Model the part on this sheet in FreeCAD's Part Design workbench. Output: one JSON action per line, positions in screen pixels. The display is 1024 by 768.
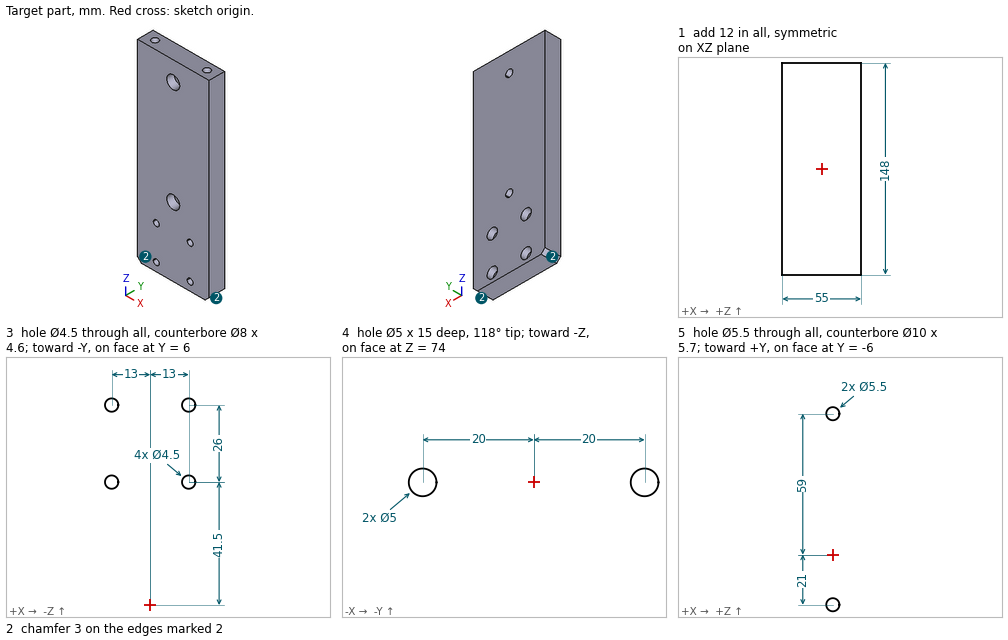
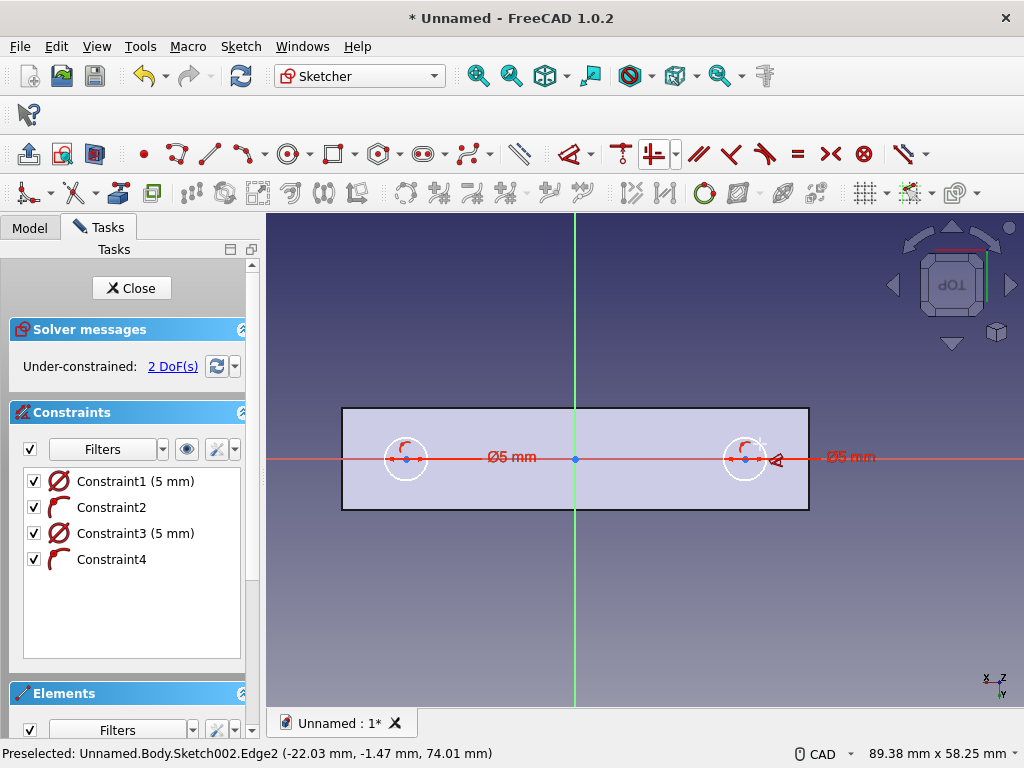
{"action": "left_click", "coordinate": [406, 459]}
{"action": "left_click", "coordinate": [491, 493]}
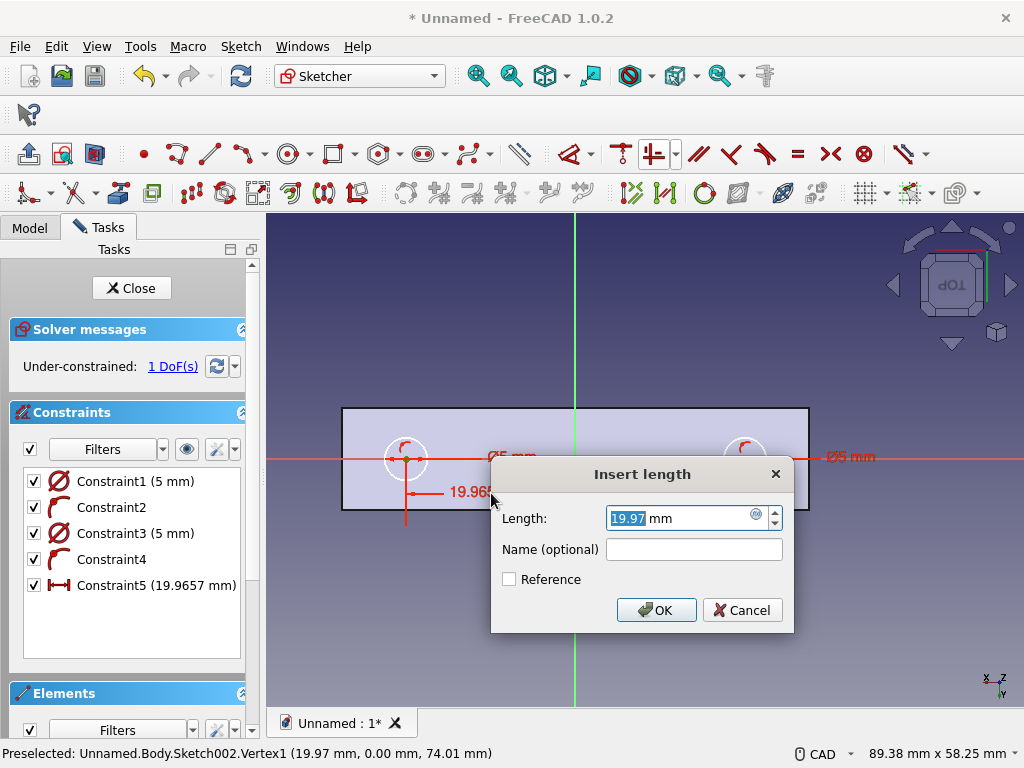
{"action": "type", "text": "20"}
{"action": "key", "text": "Return"}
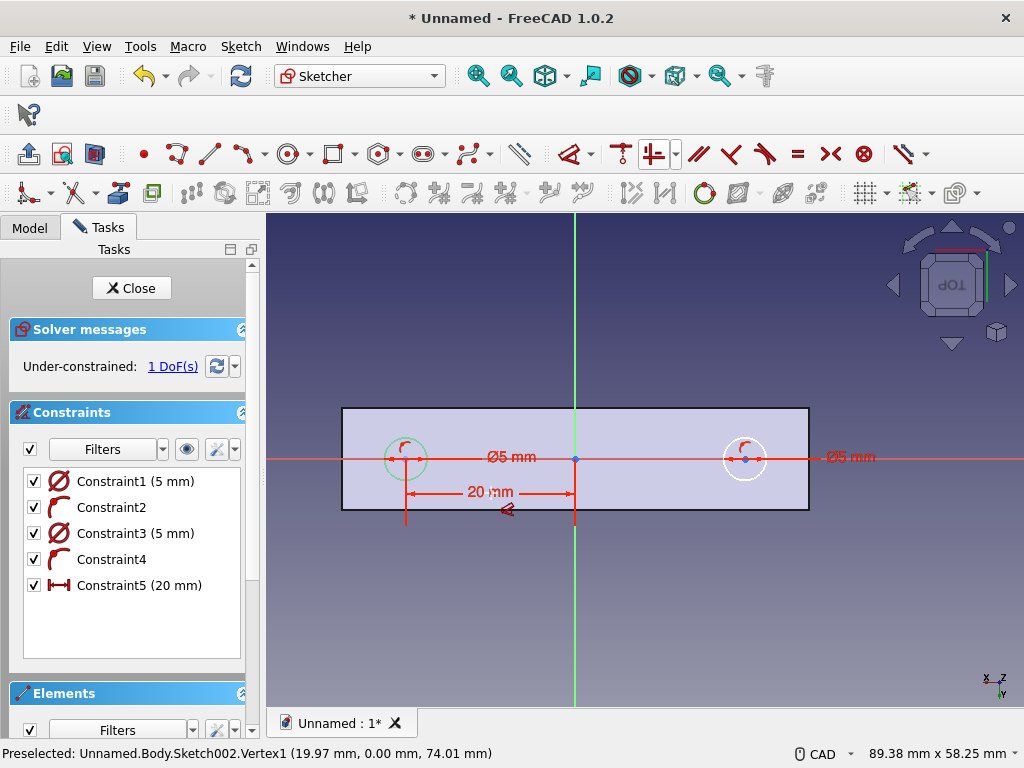
{"action": "left_click", "coordinate": [745, 459]}
{"action": "left_click", "coordinate": [660, 493]}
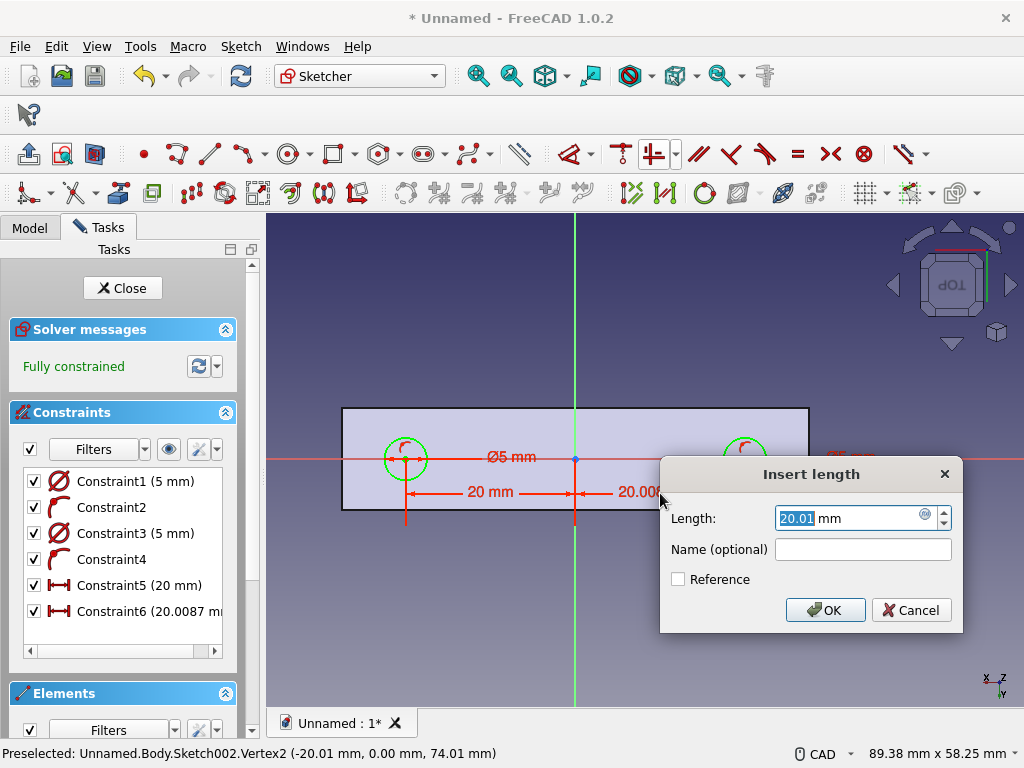
{"action": "type", "text": "20"}
{"action": "key", "text": "Return"}
{"action": "key", "text": "Escape"}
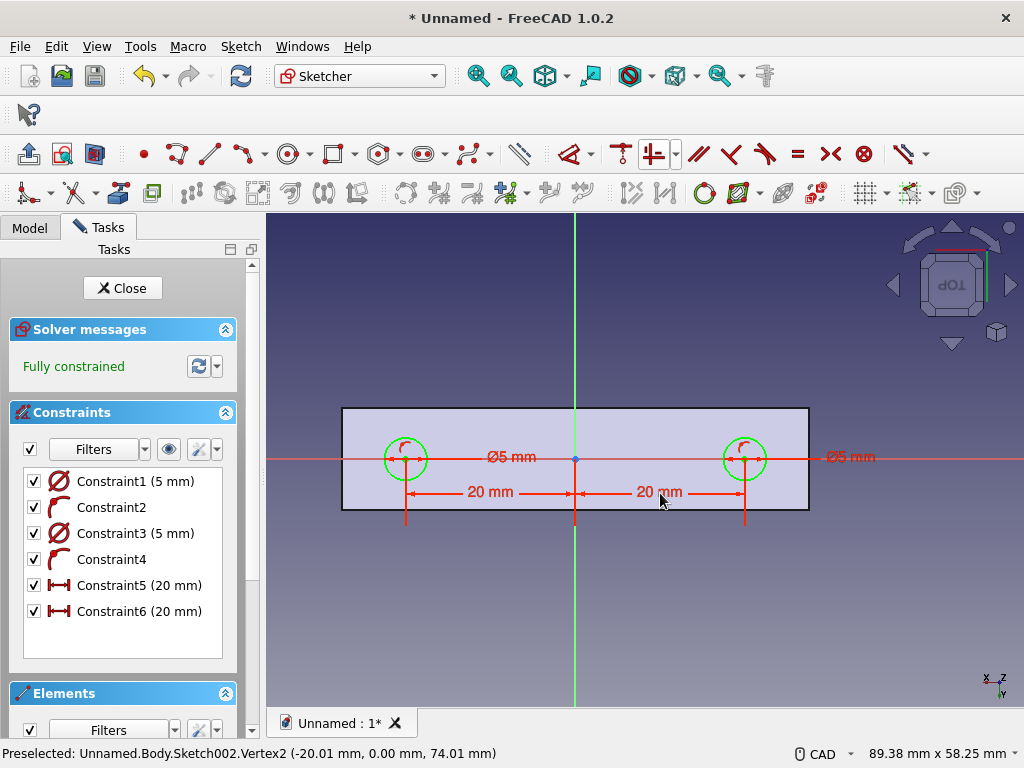
{"action": "left_click", "coordinate": [123, 288]}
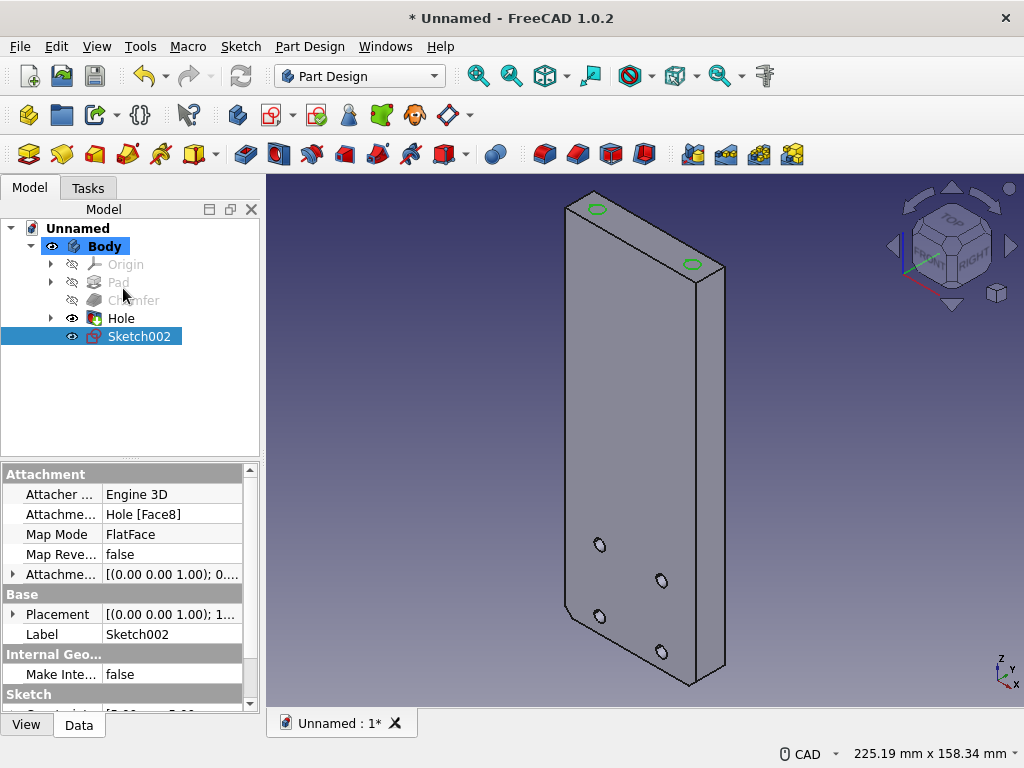
{"action": "left_click", "coordinate": [279, 154]}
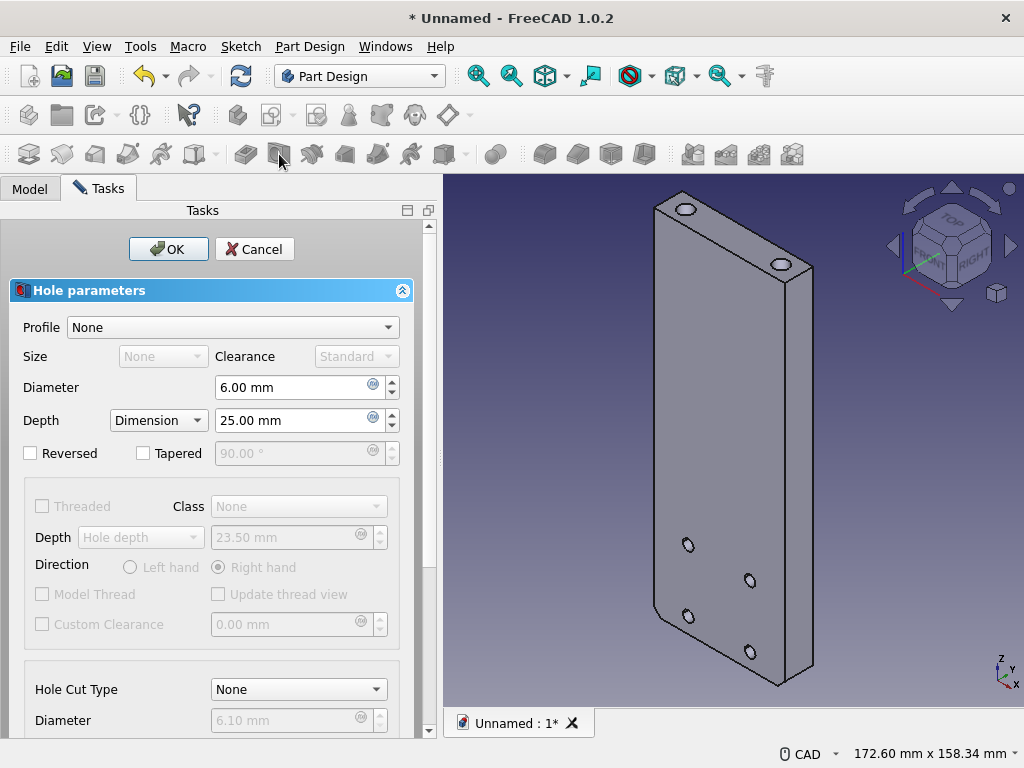
{"action": "triple_click", "coordinate": [300, 388]}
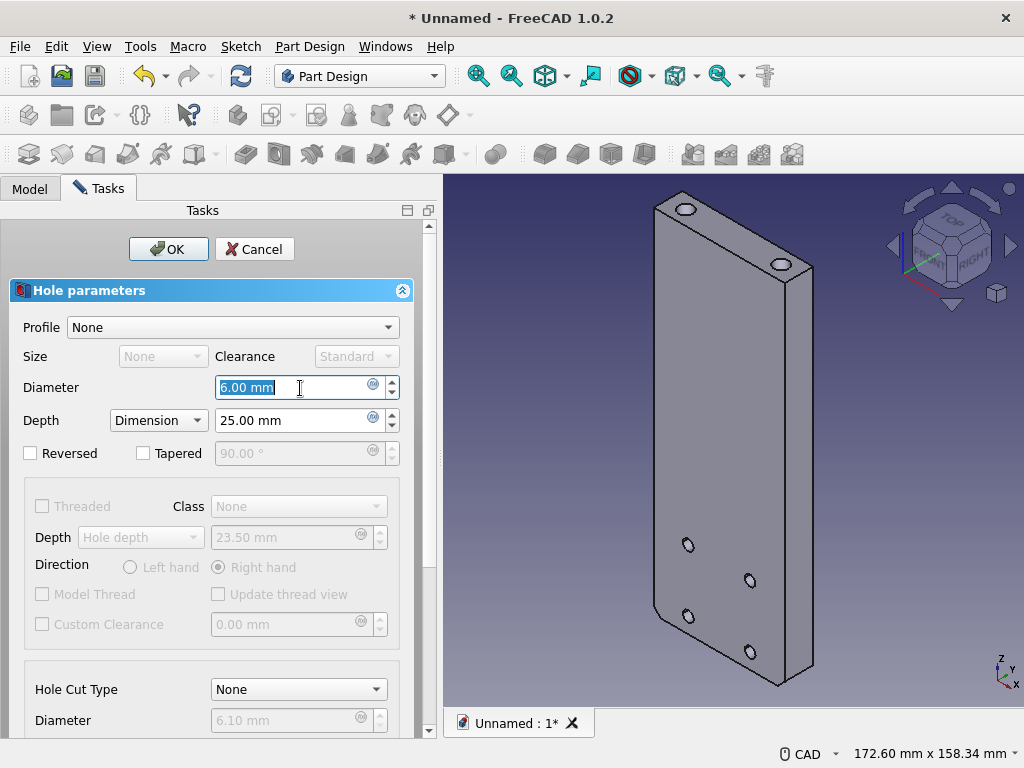
{"action": "type", "text": "5"}
{"action": "key", "text": "Tab"}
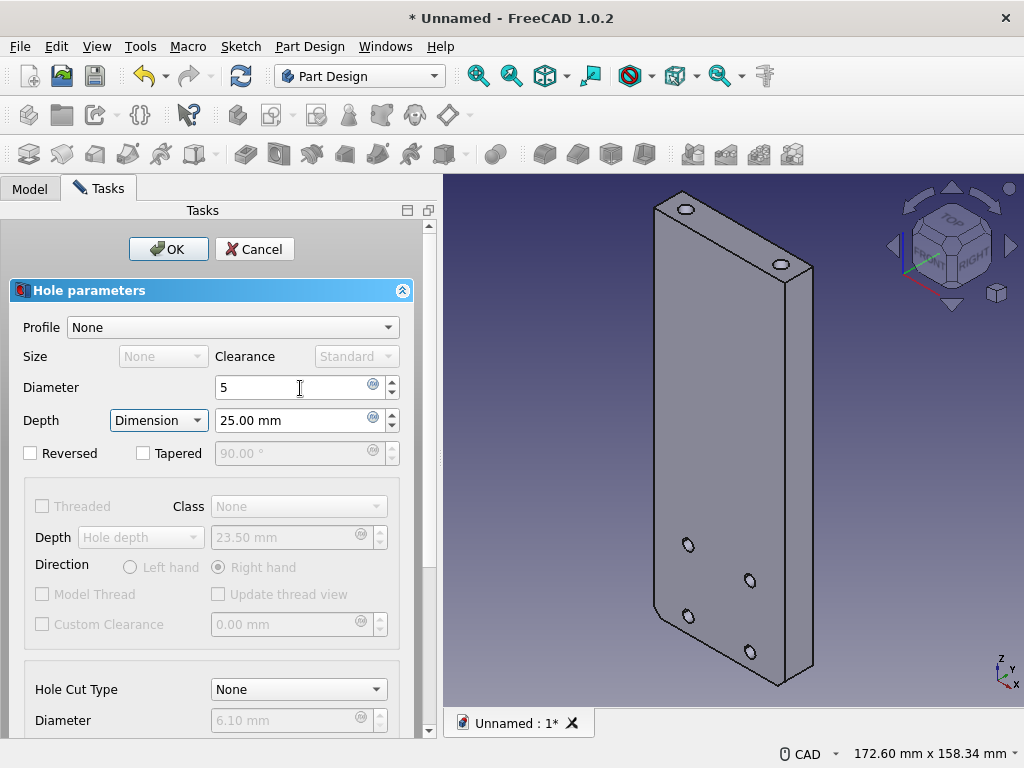
{"action": "triple_click", "coordinate": [300, 420]}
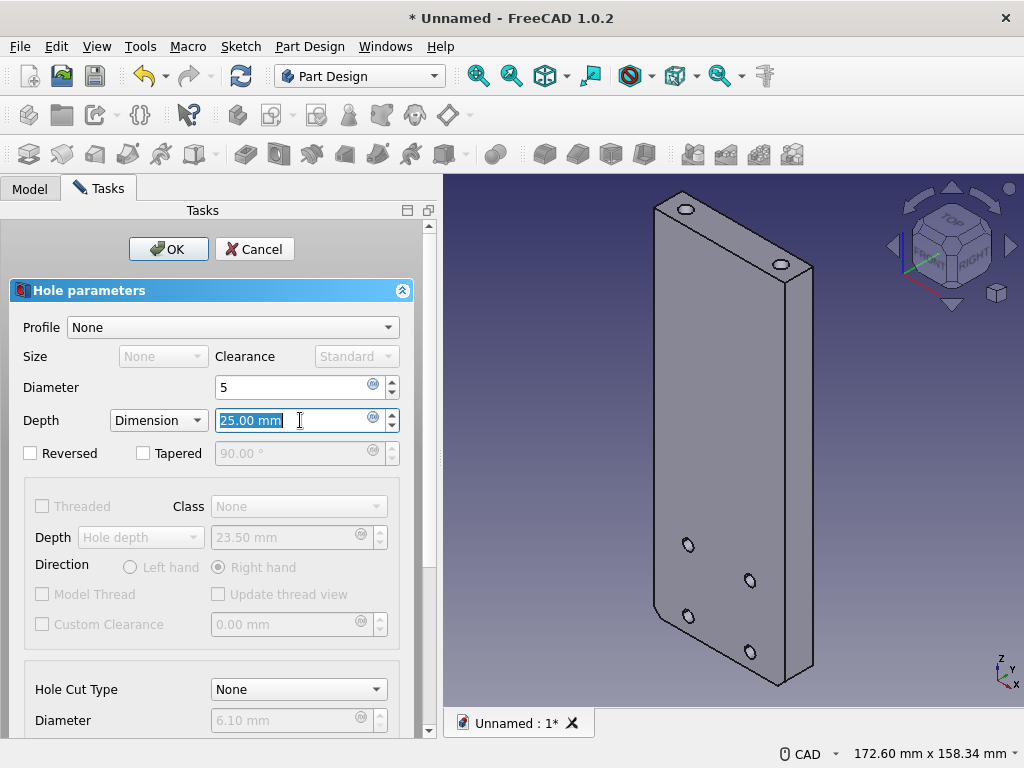
{"action": "type", "text": "15"}
{"action": "key", "text": "Tab"}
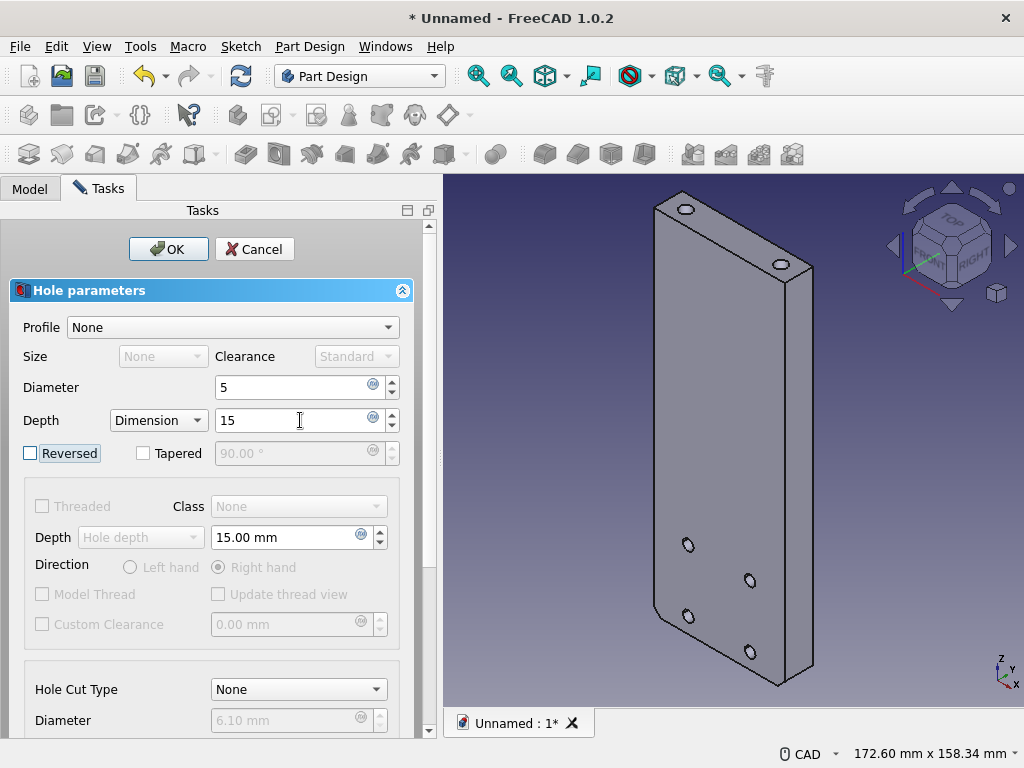
{"action": "left_click", "coordinate": [169, 249]}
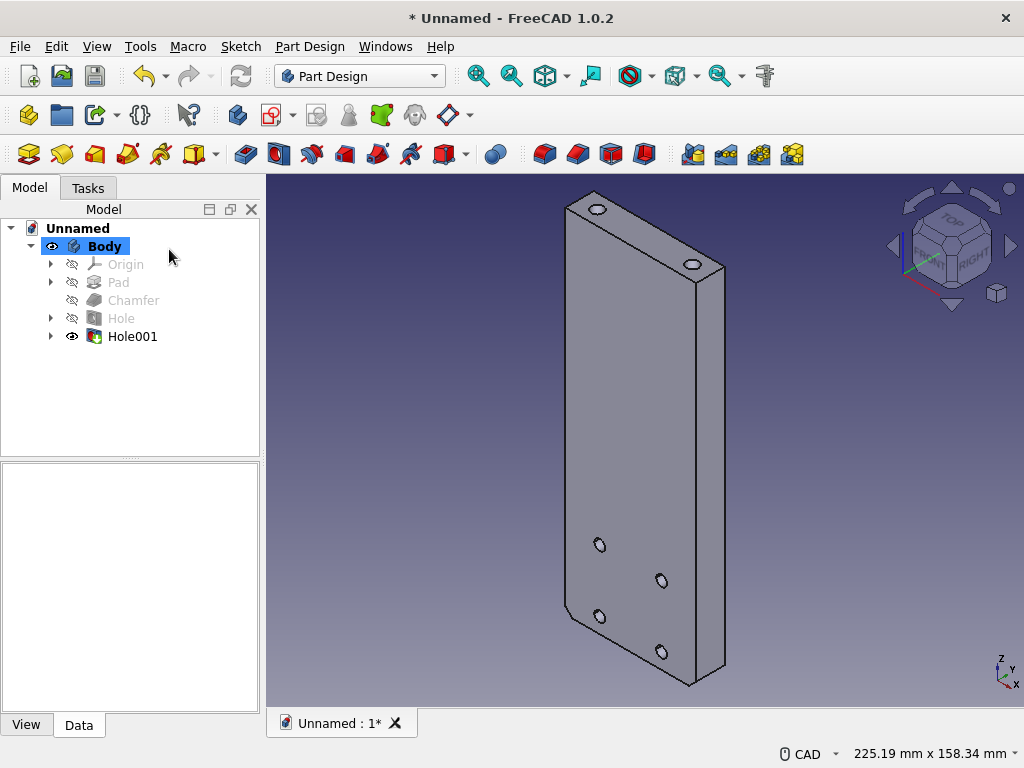
{"action": "left_click", "coordinate": [631, 332]}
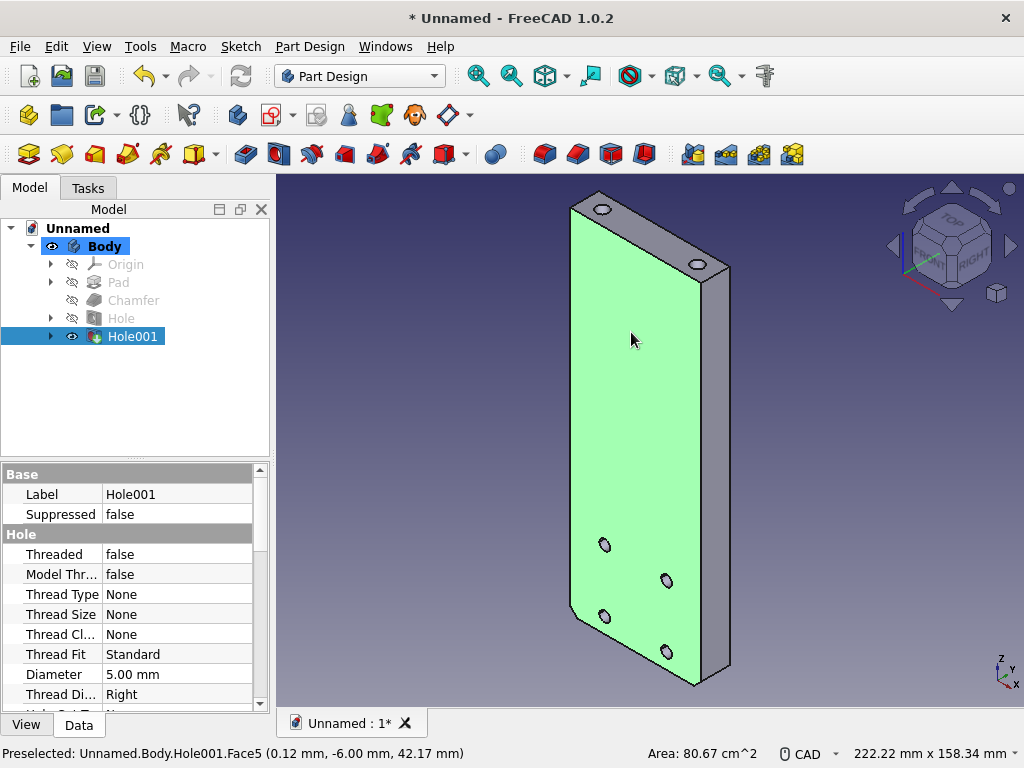
{"action": "left_click", "coordinate": [270, 116]}